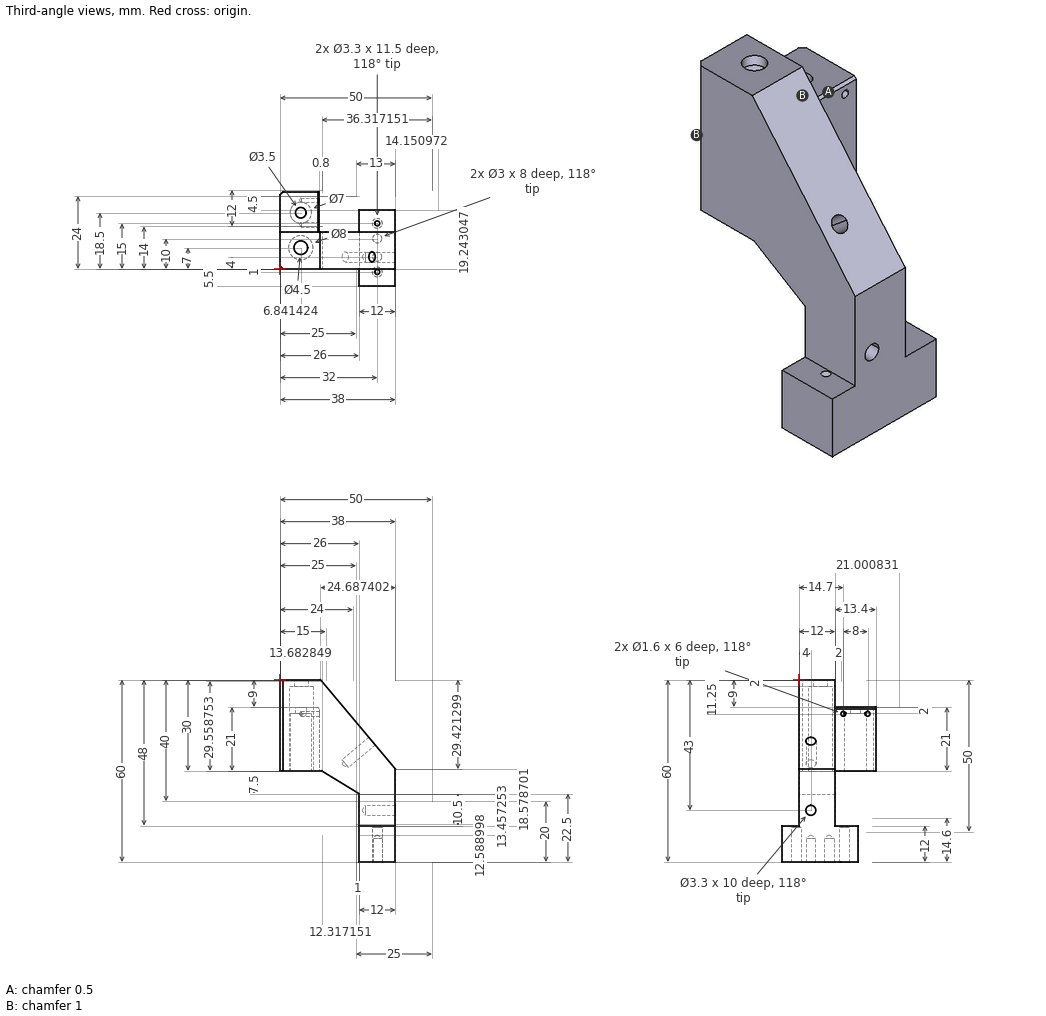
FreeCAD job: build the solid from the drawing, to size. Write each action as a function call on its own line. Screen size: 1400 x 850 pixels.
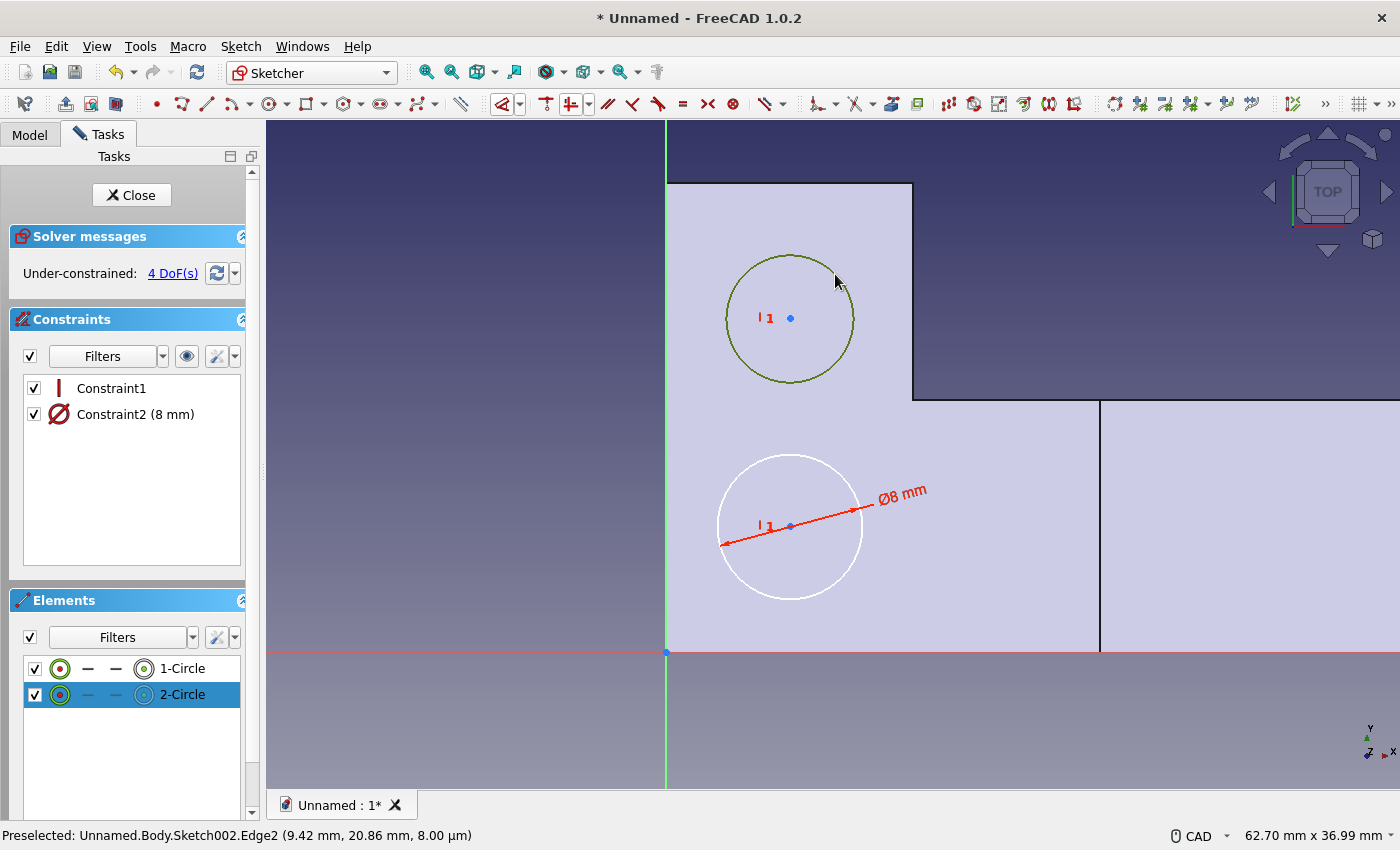
click(520, 104)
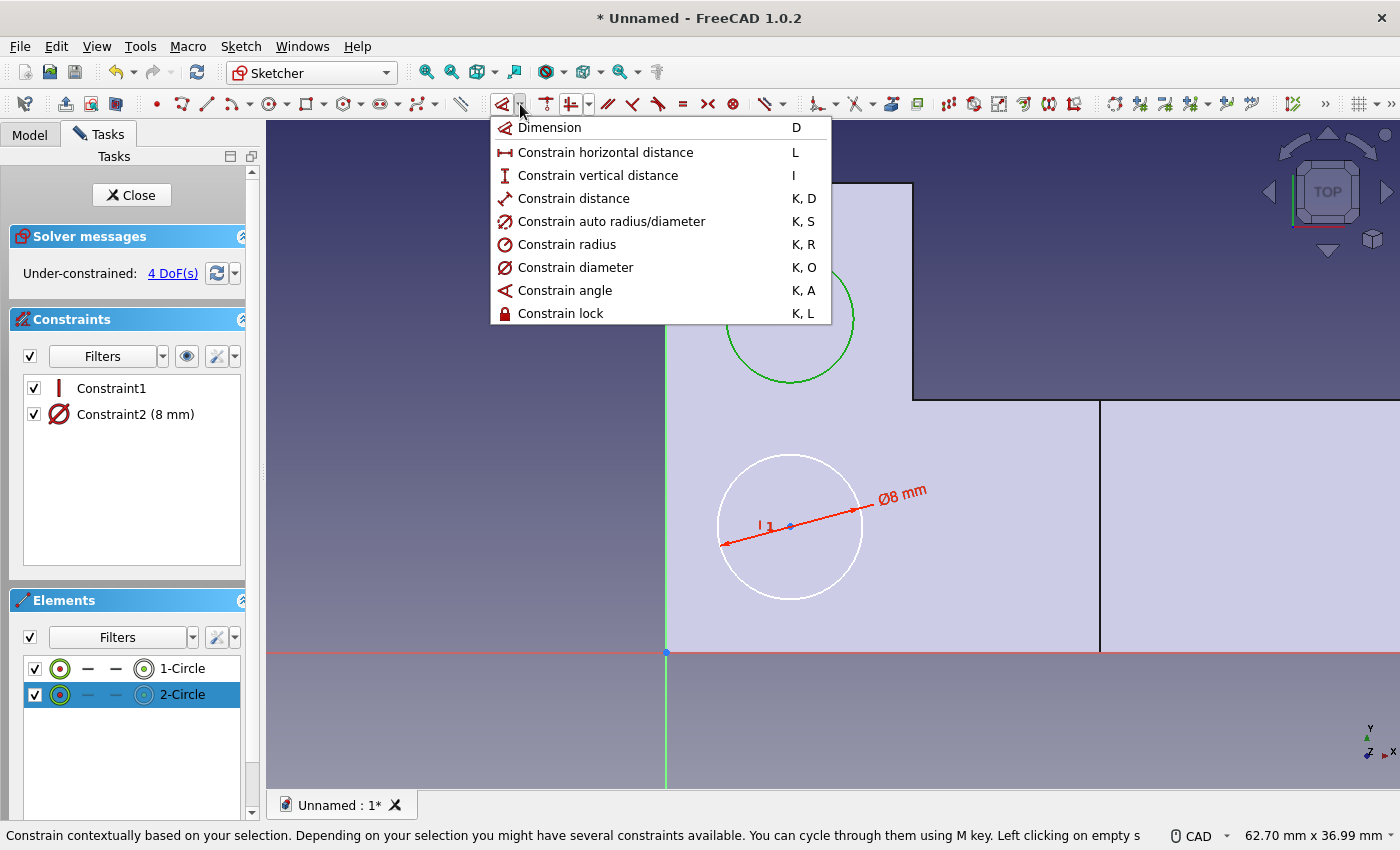
click(661, 268)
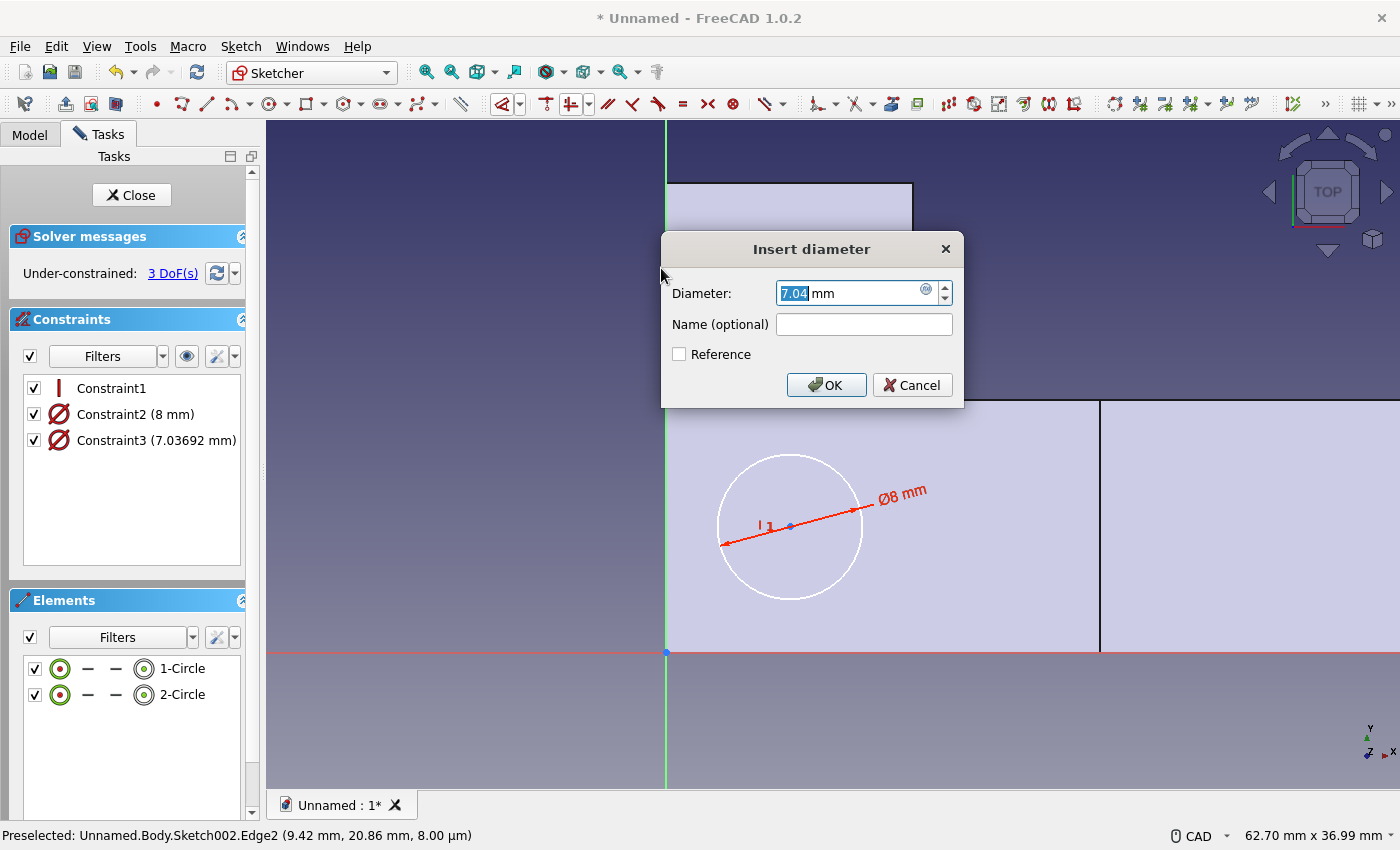
text(7)
key(Return)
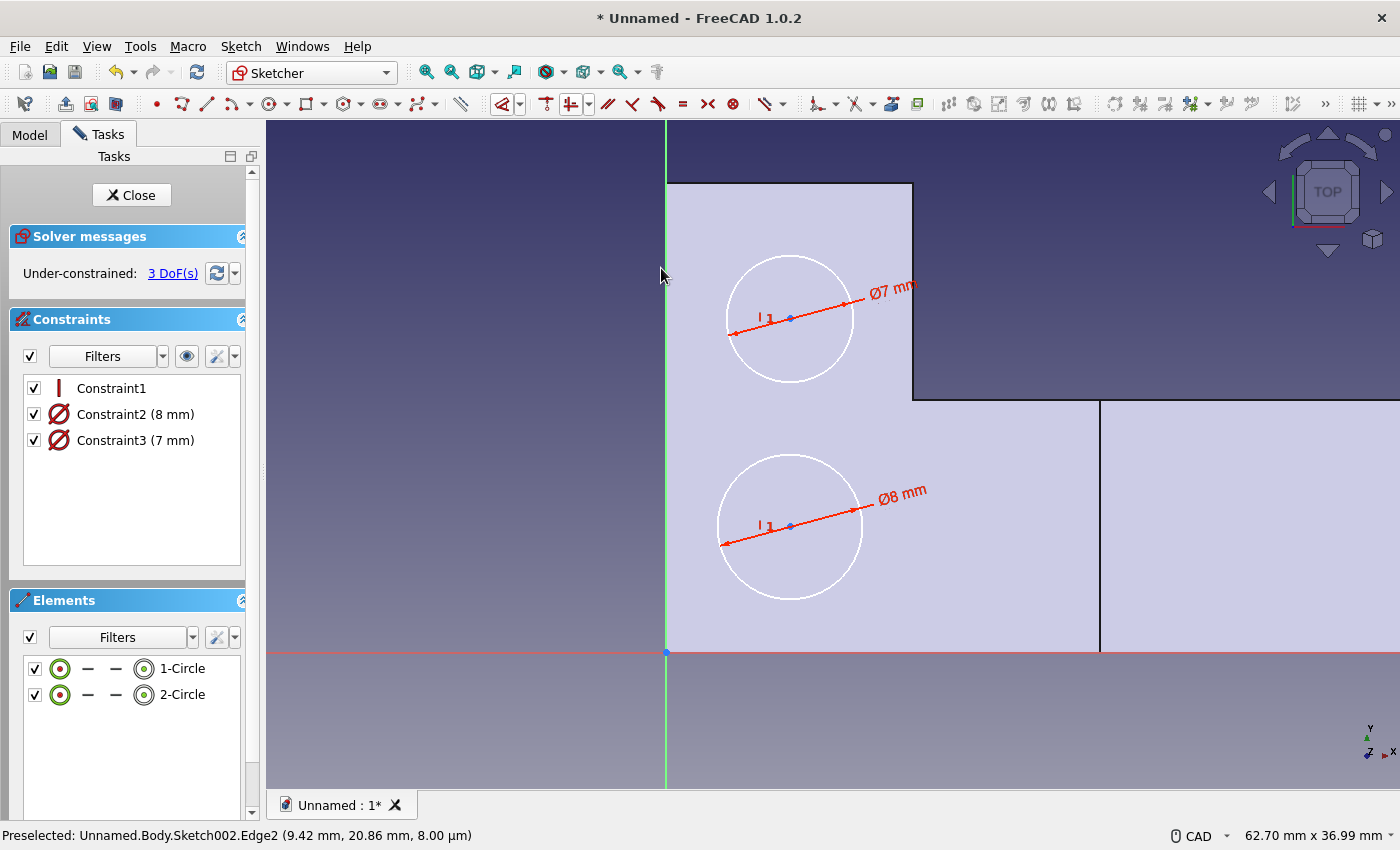
click(790, 527)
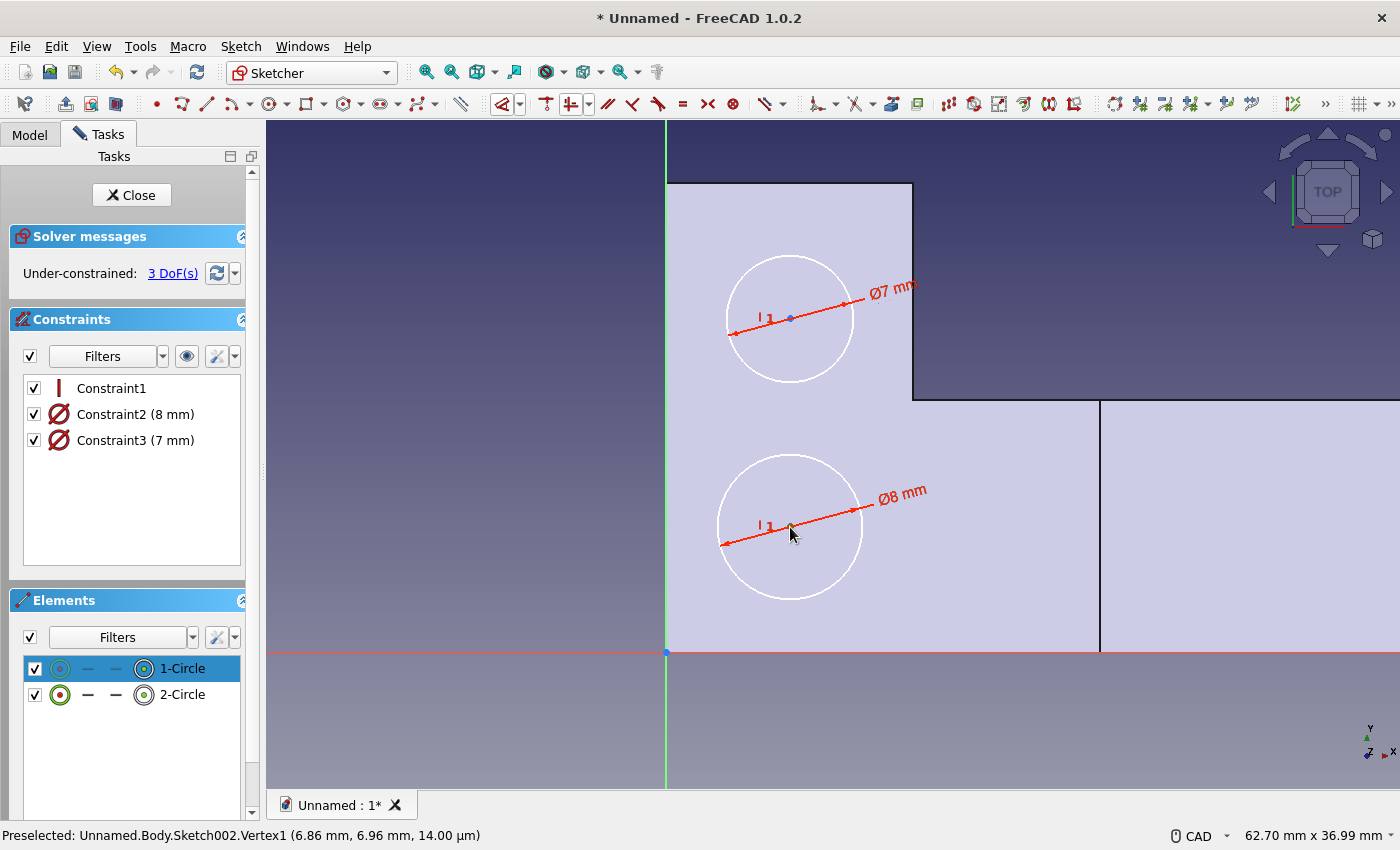
key(i)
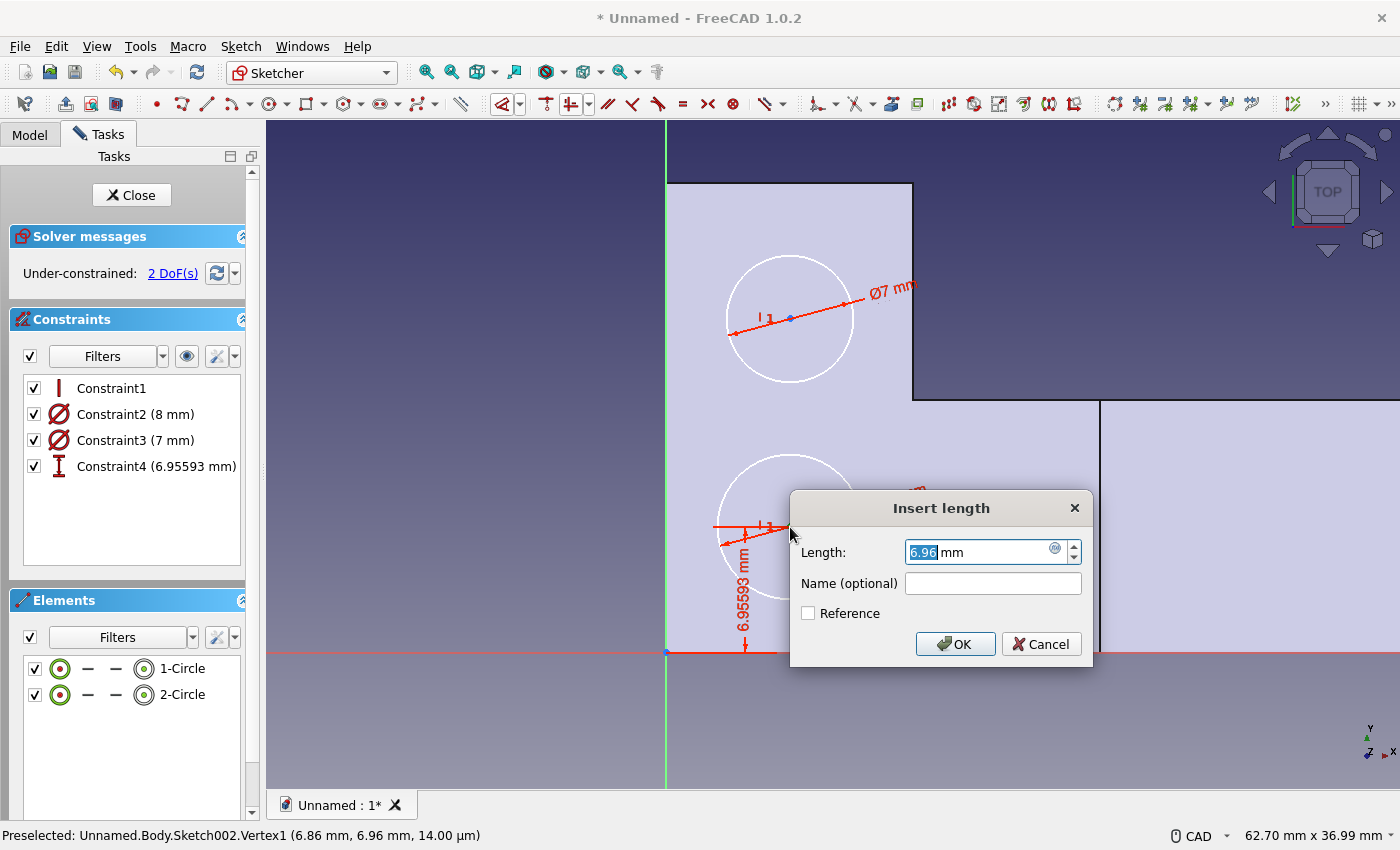
text(7)
key(Return)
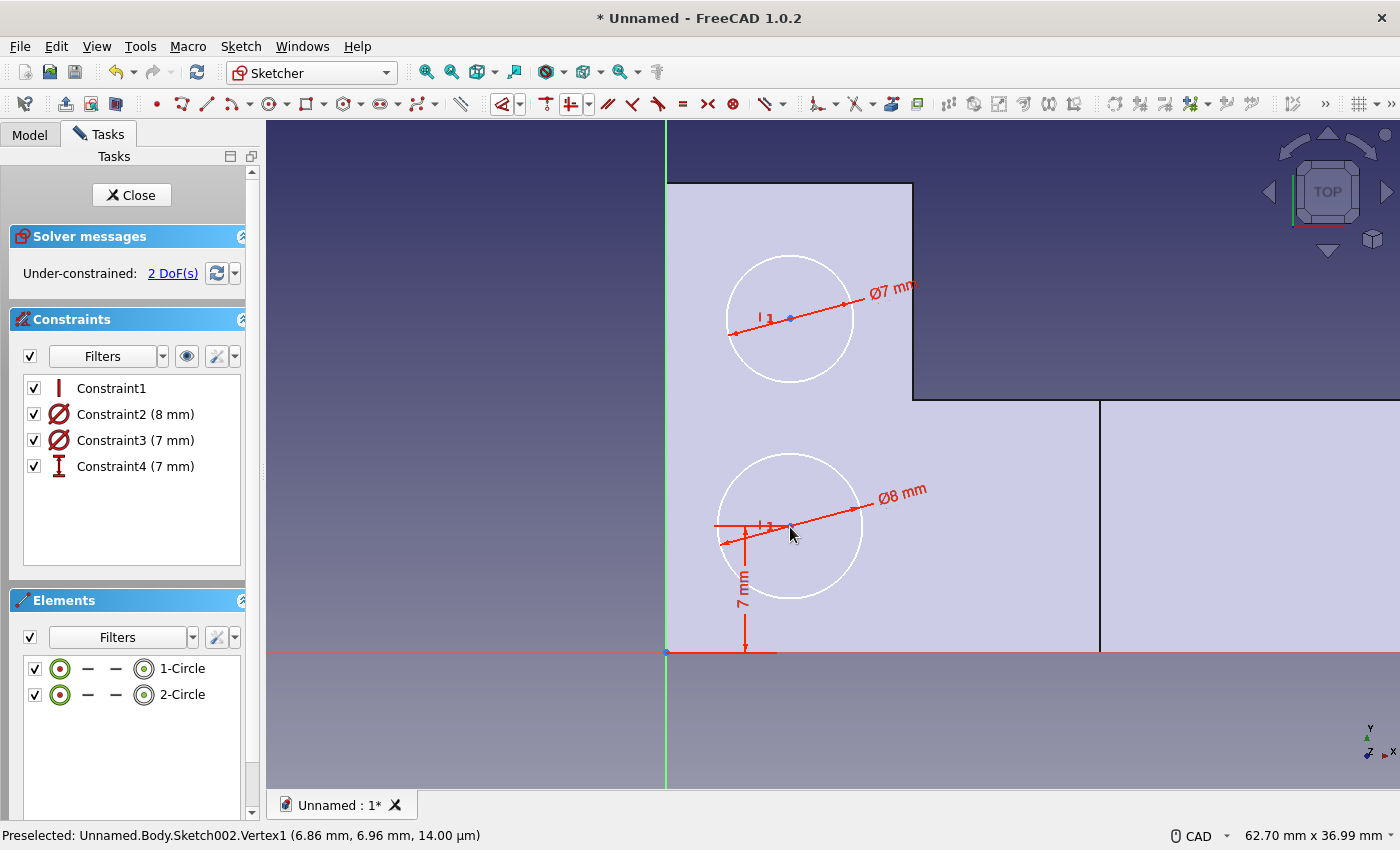
click(790, 319)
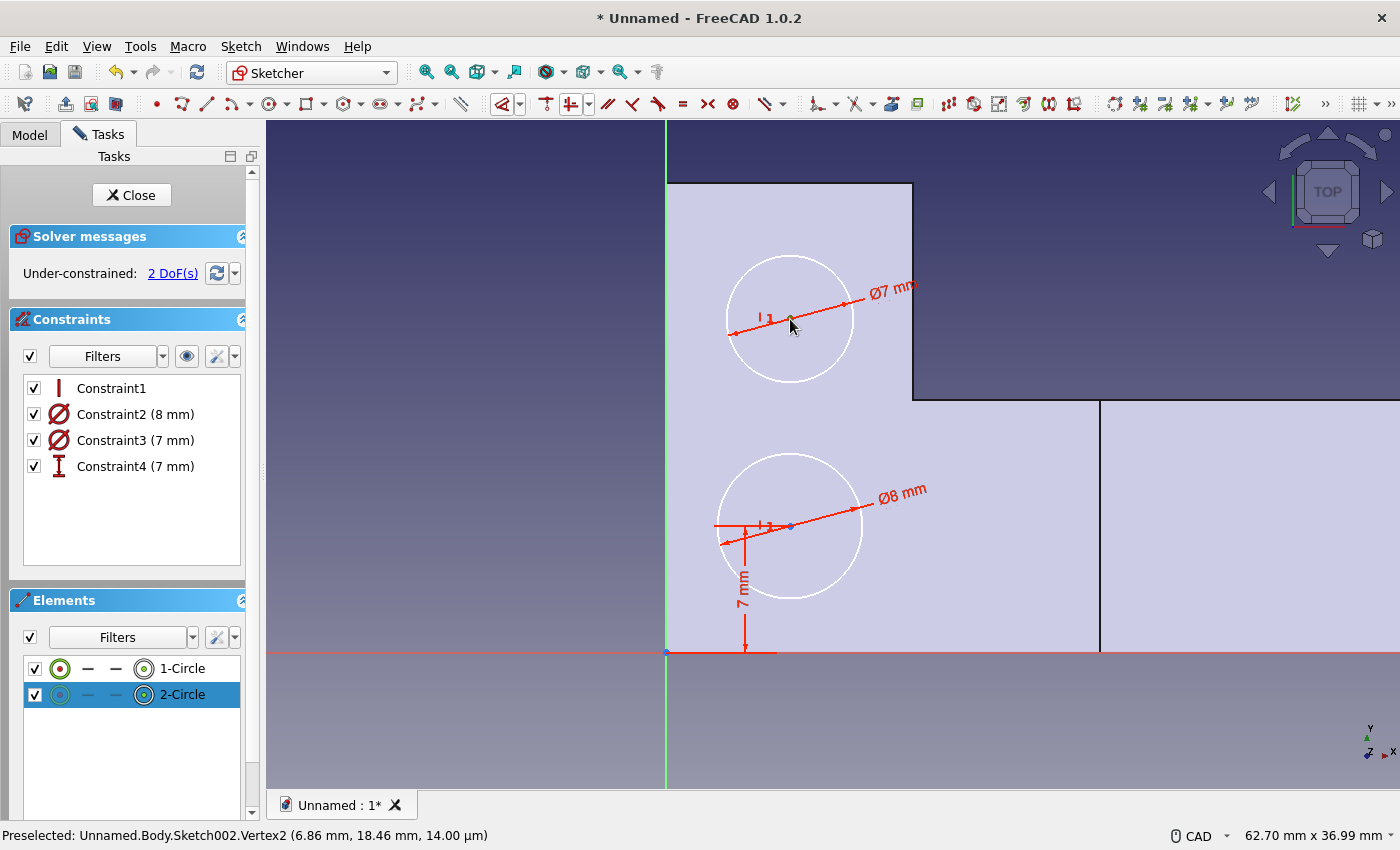
click(520, 104)